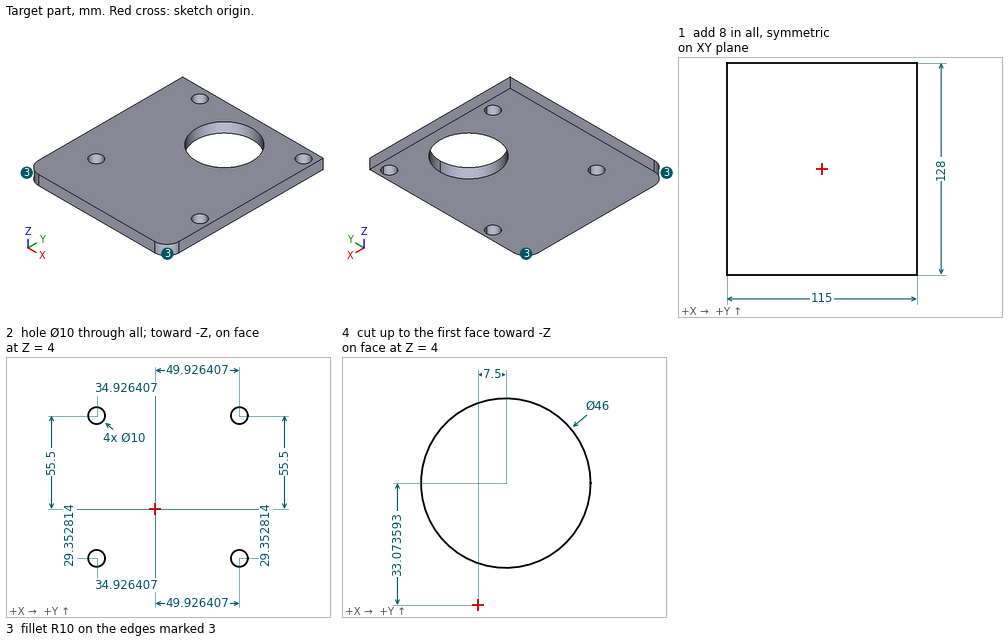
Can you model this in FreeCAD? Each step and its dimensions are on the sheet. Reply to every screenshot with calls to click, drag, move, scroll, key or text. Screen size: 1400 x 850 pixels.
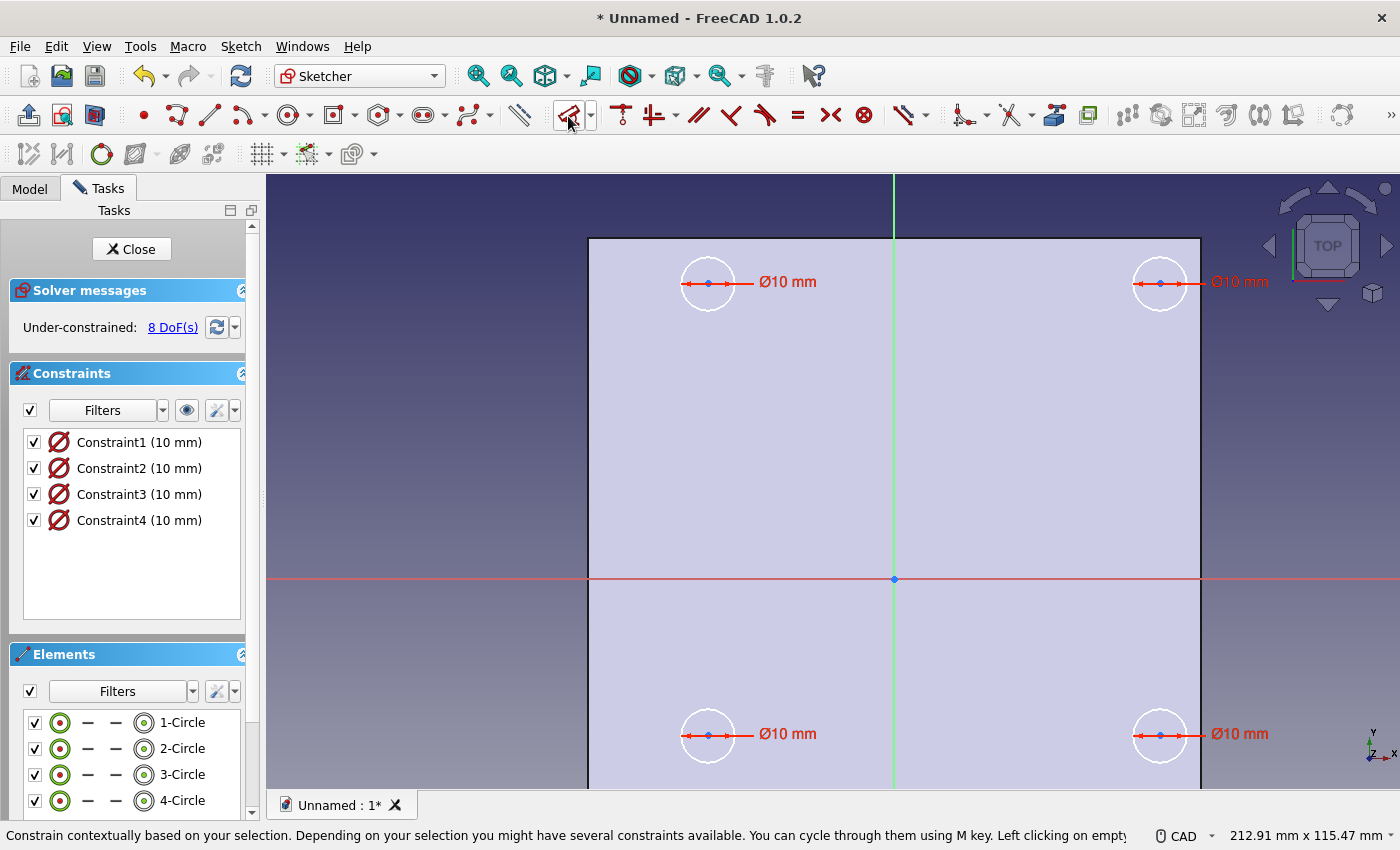
click(708, 284)
click(674, 432)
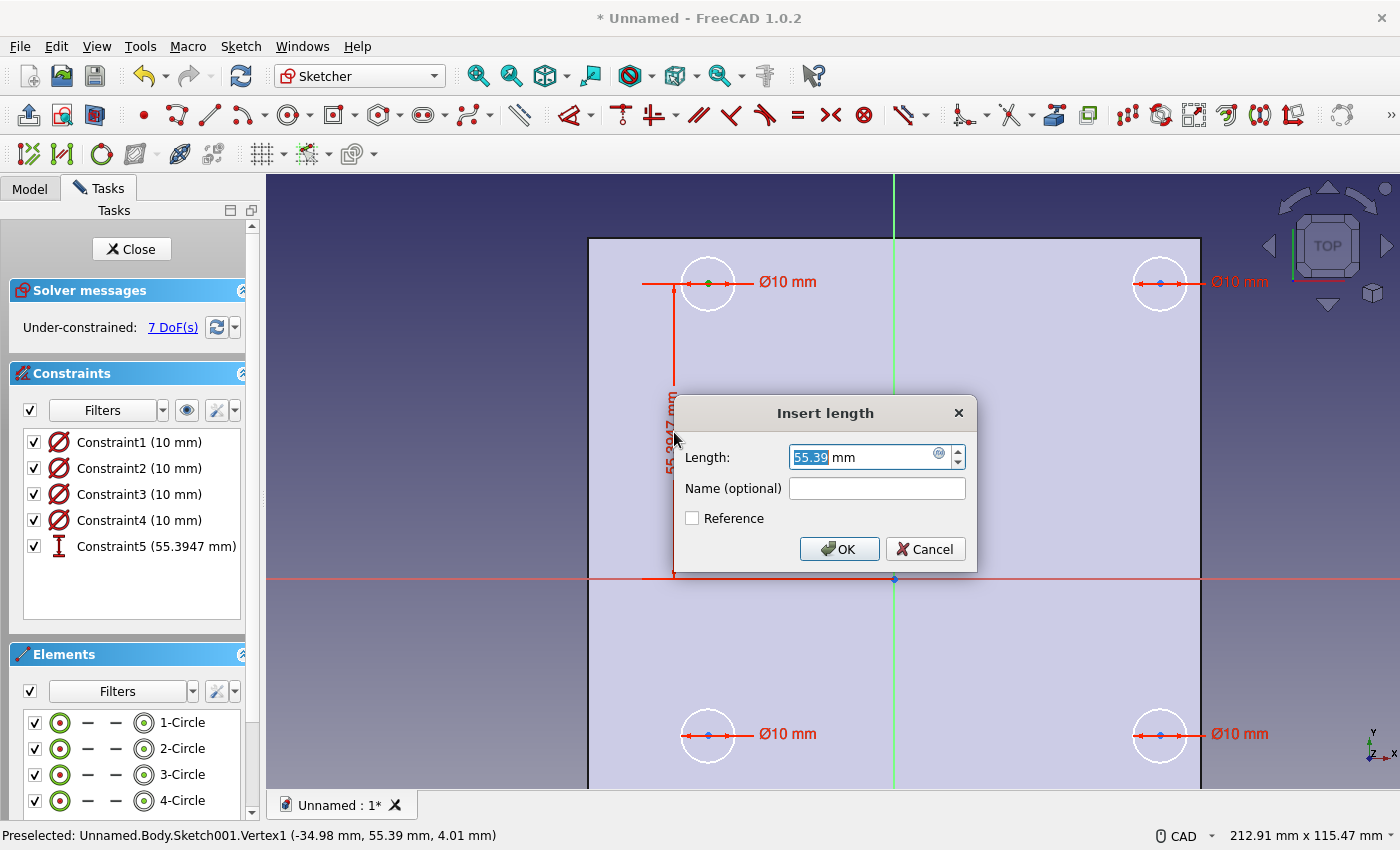
text(55.5)
key(Return)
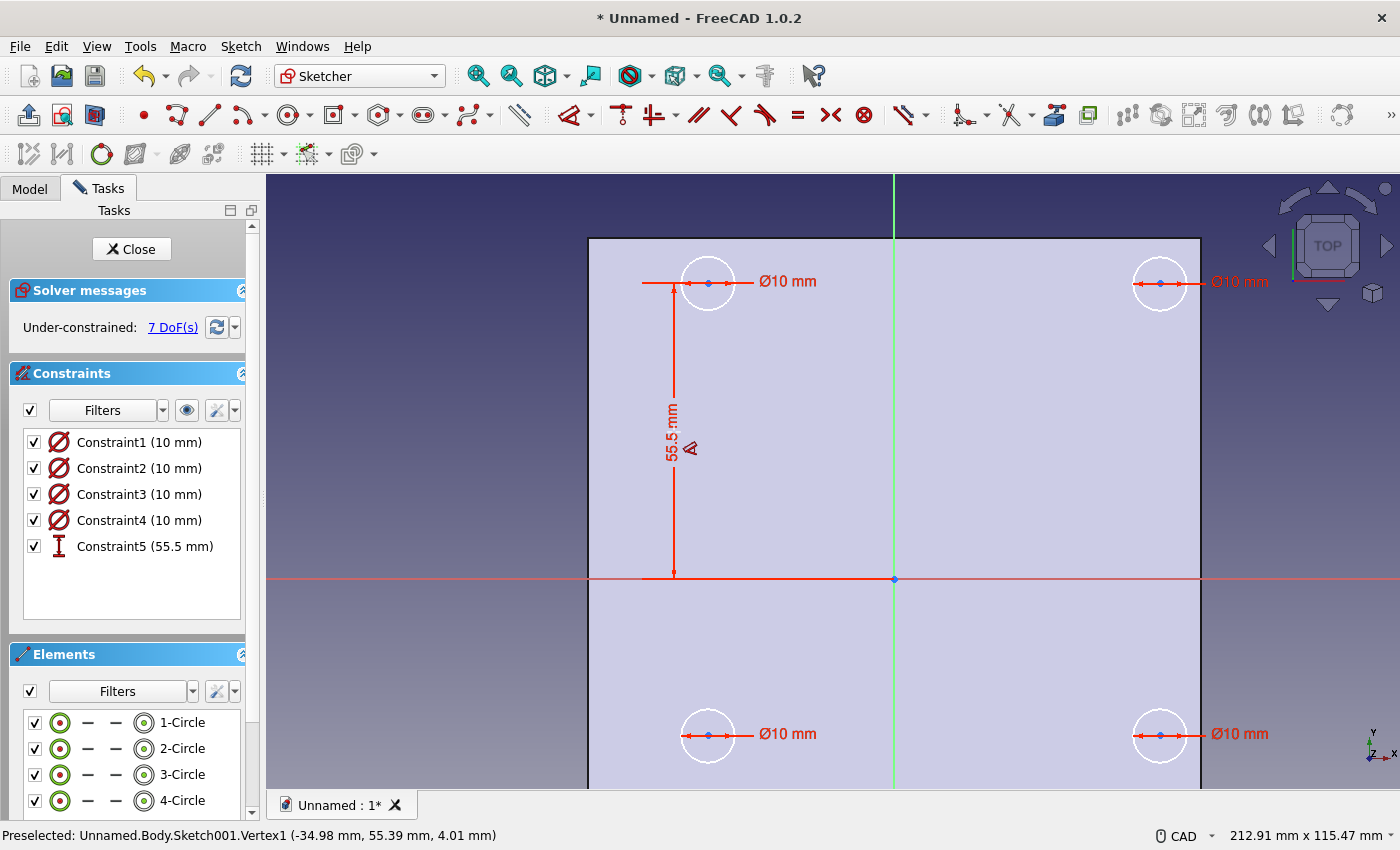
click(1160, 284)
click(1194, 432)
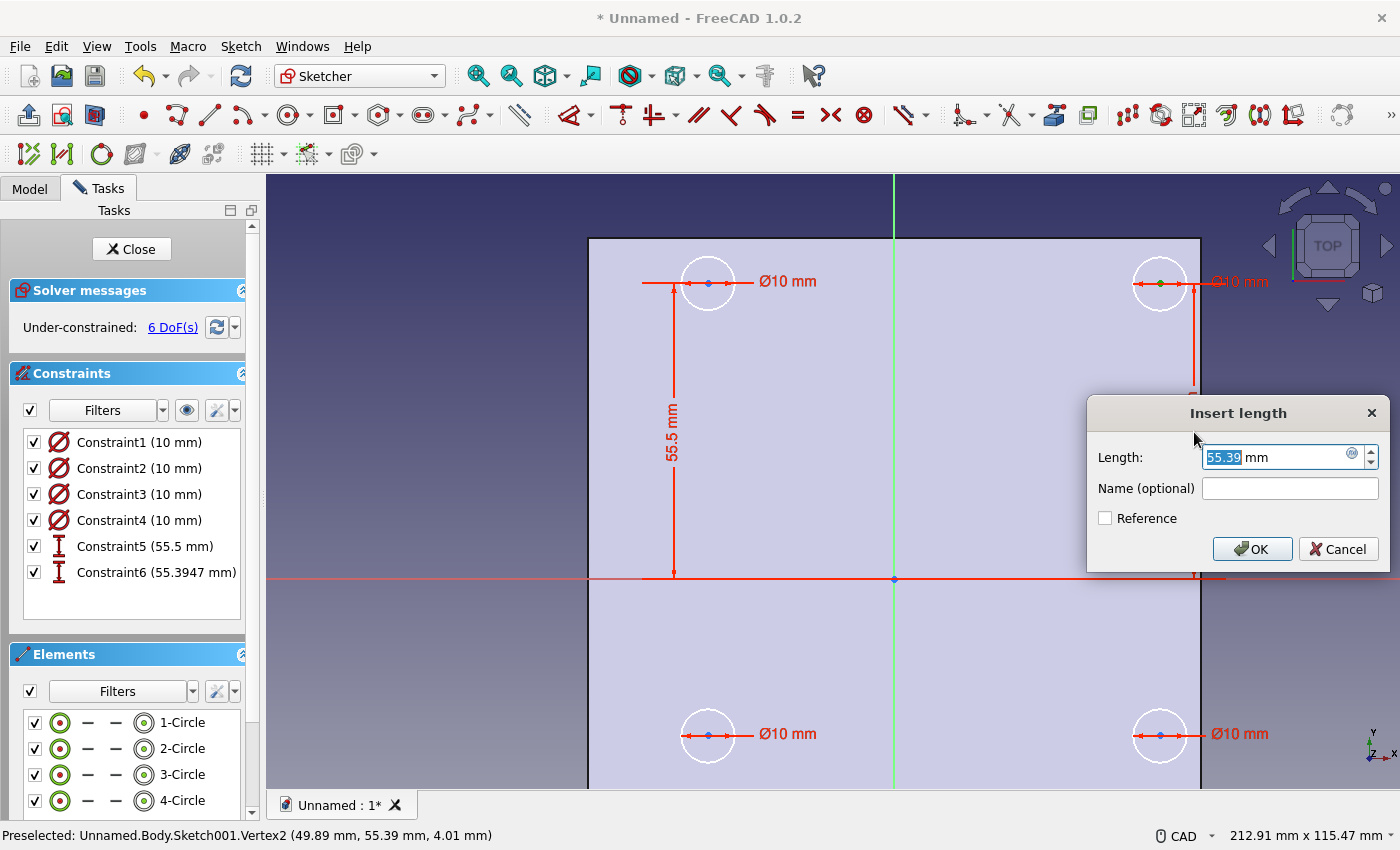
text(55.5)
key(Return)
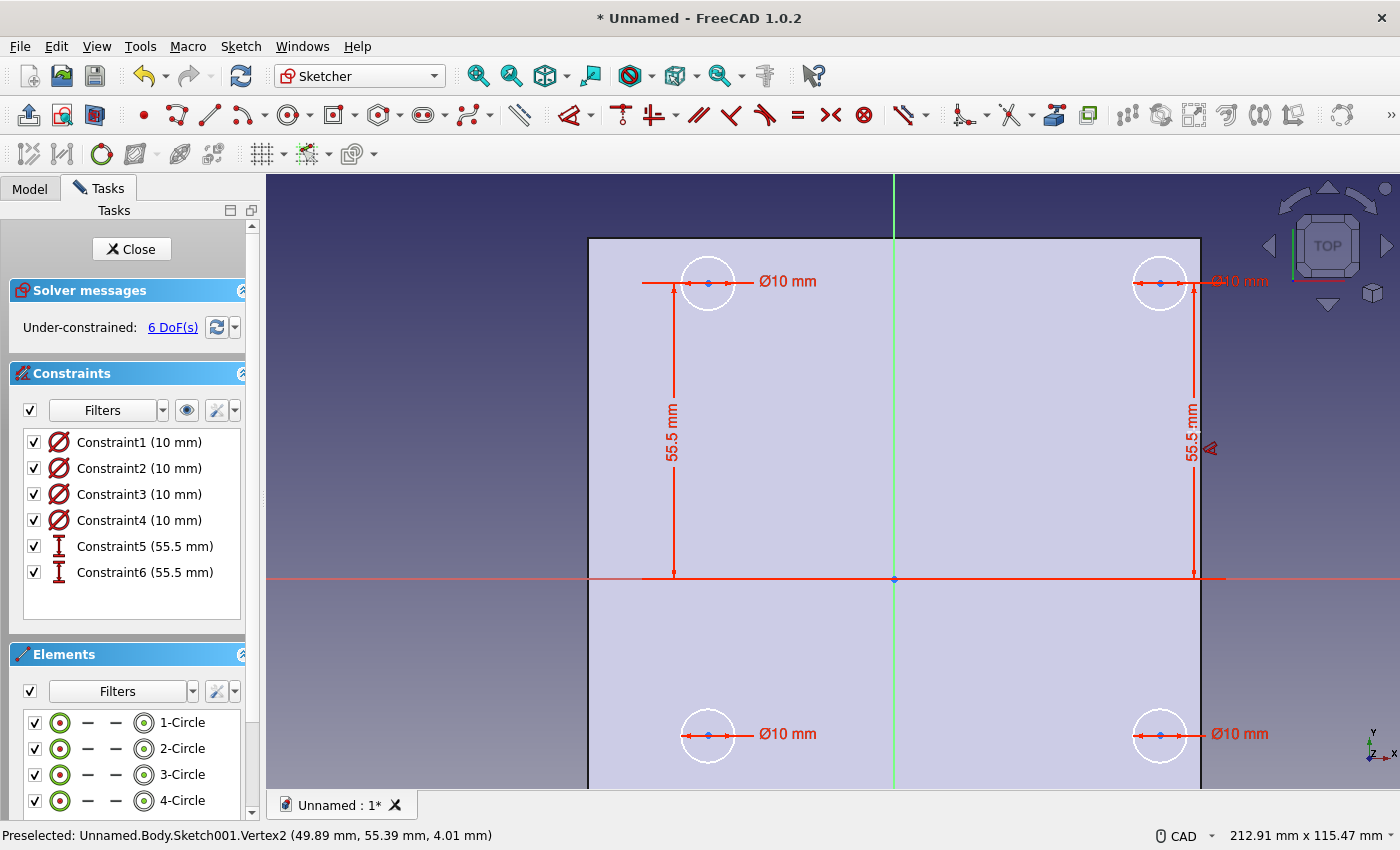
click(708, 283)
click(801, 249)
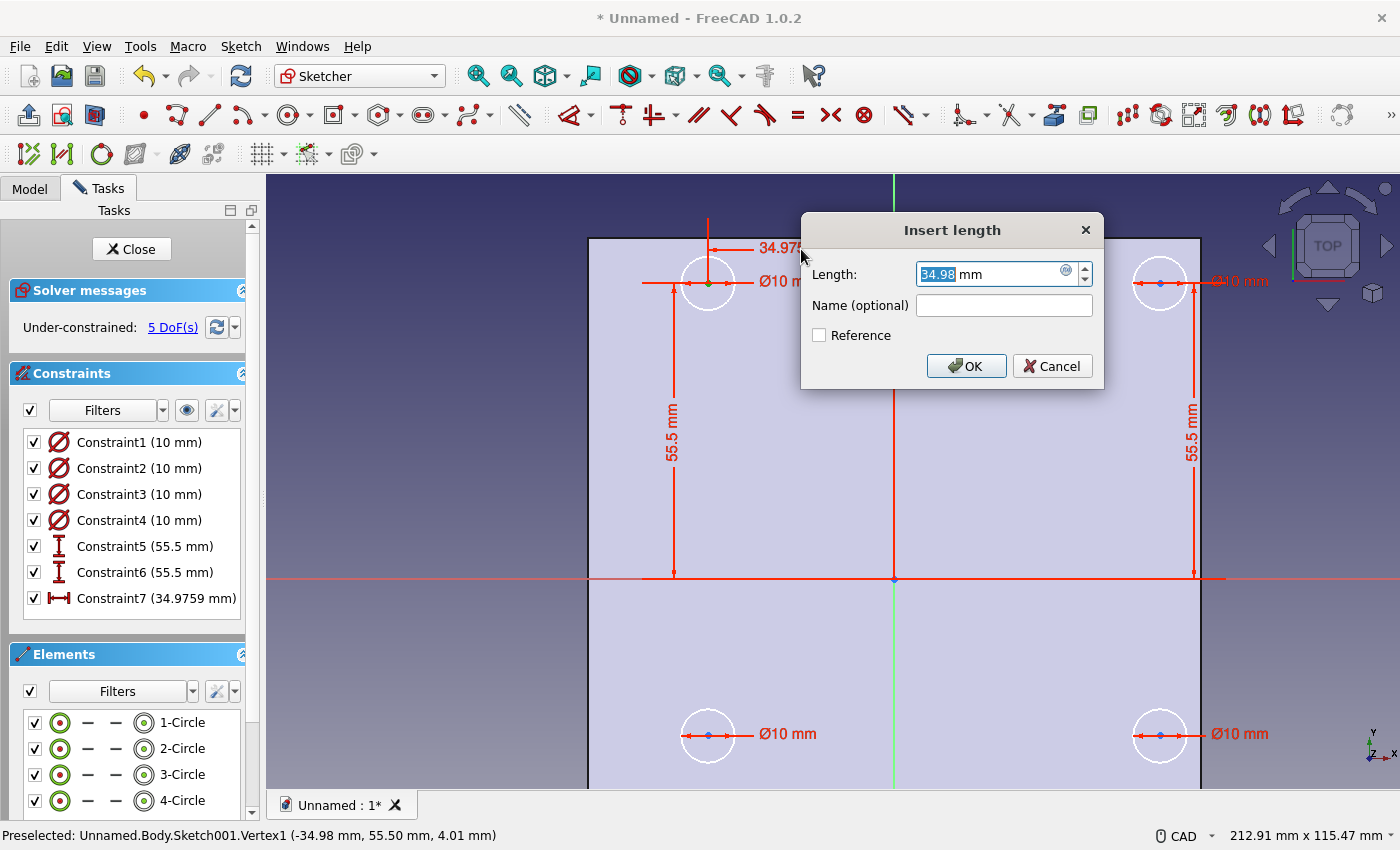
text(34.926407)
key(Return)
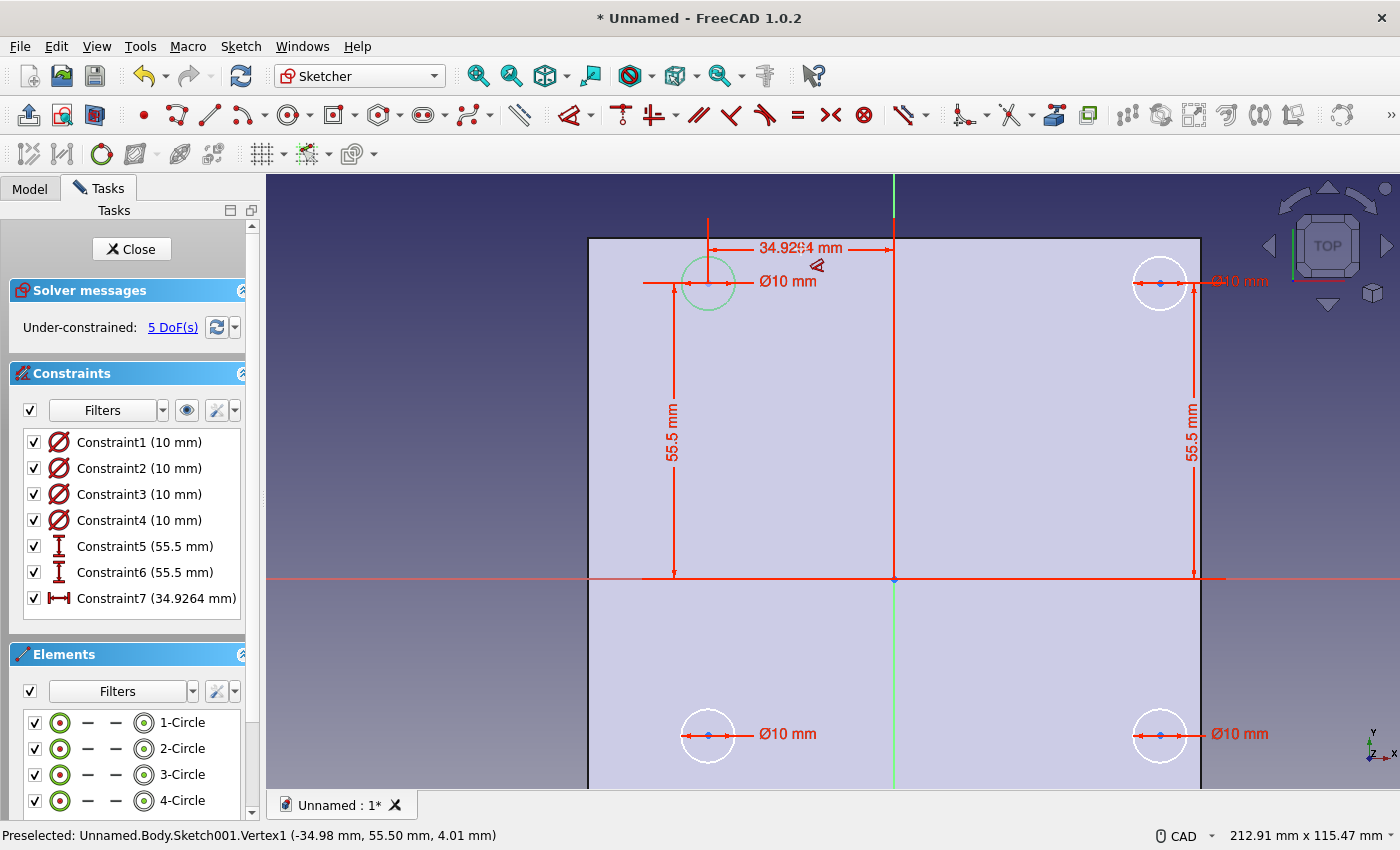
click(1160, 283)
click(1027, 249)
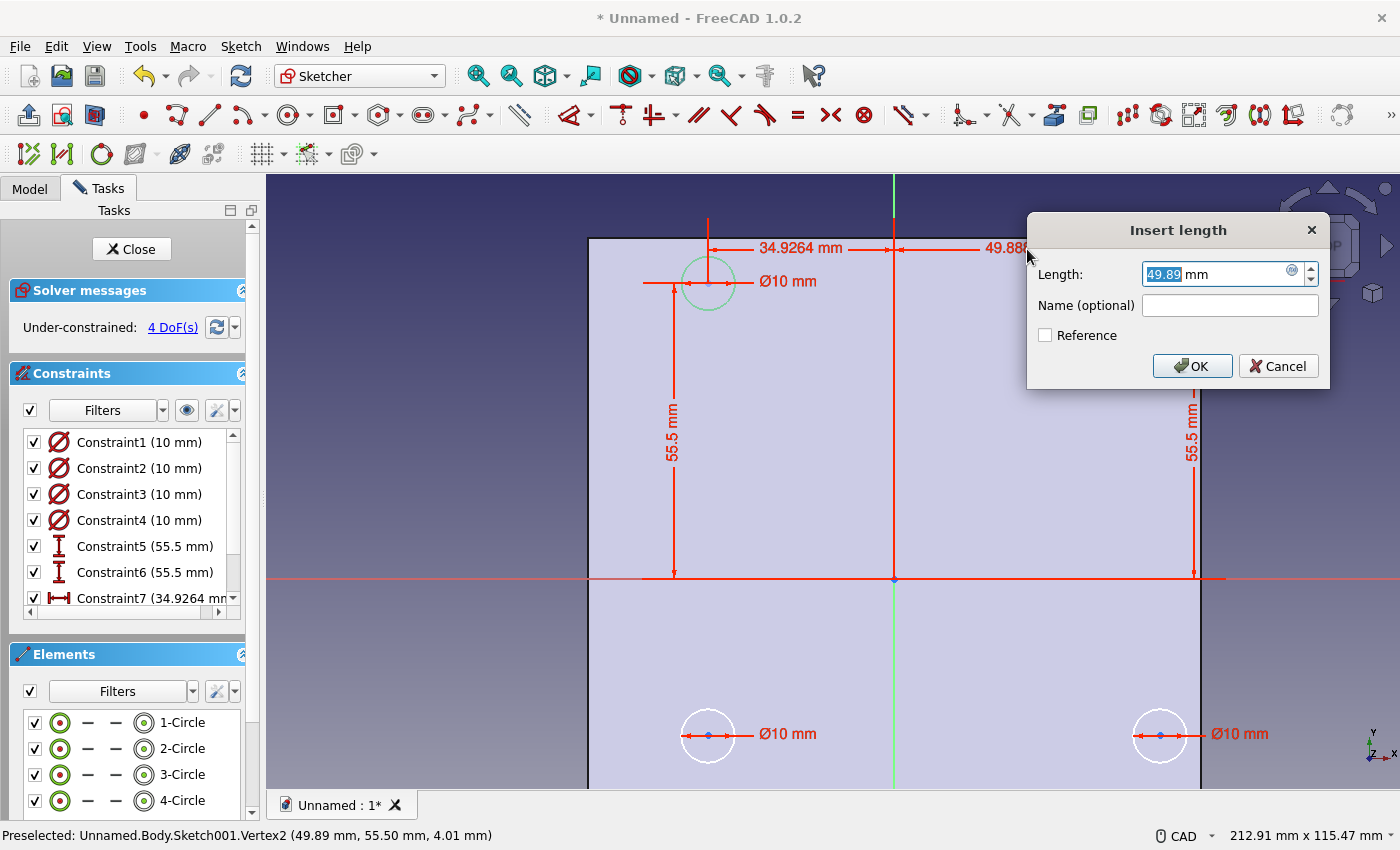
text(49.926407)
key(Return)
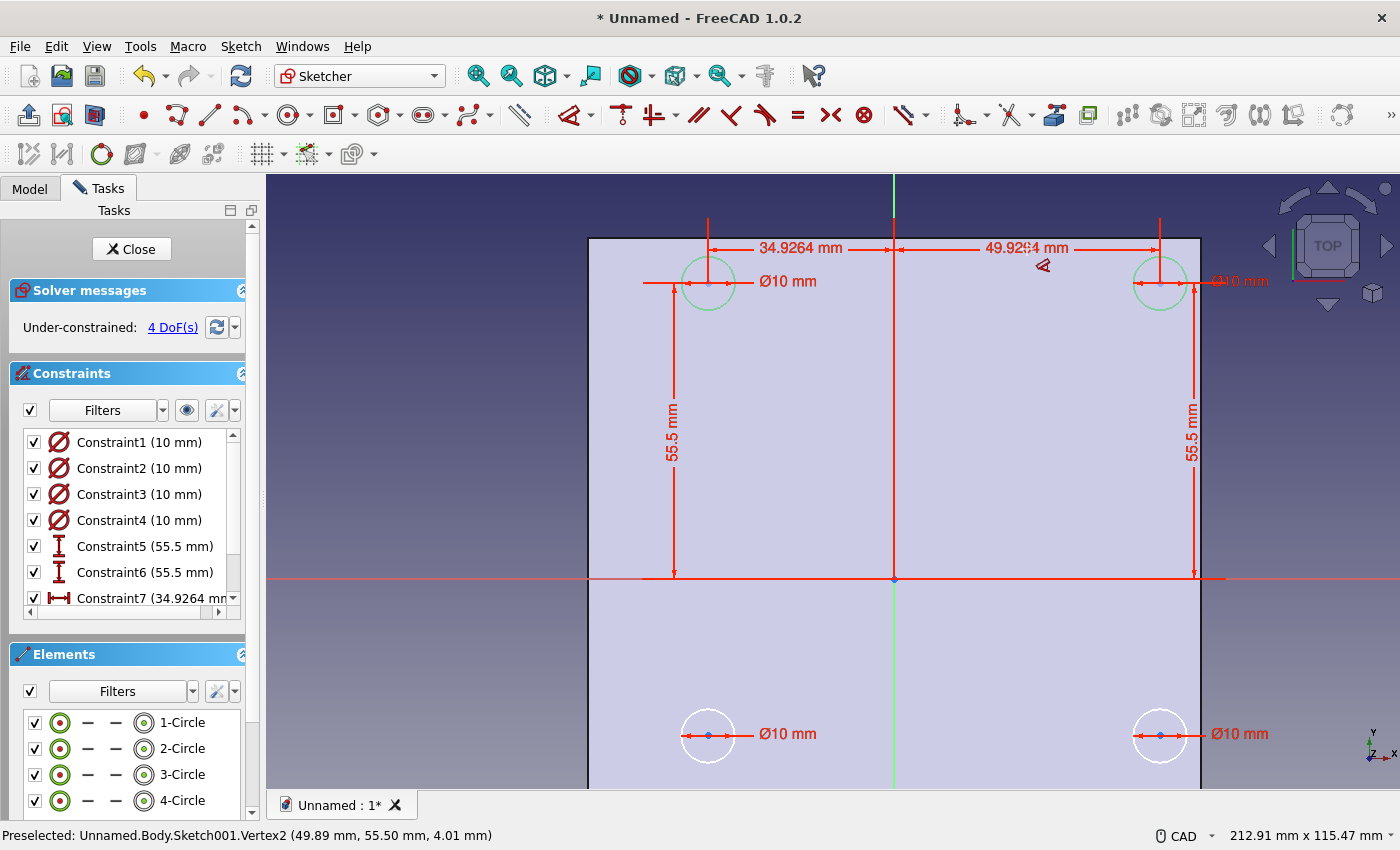
click(1160, 736)
click(1027, 545)